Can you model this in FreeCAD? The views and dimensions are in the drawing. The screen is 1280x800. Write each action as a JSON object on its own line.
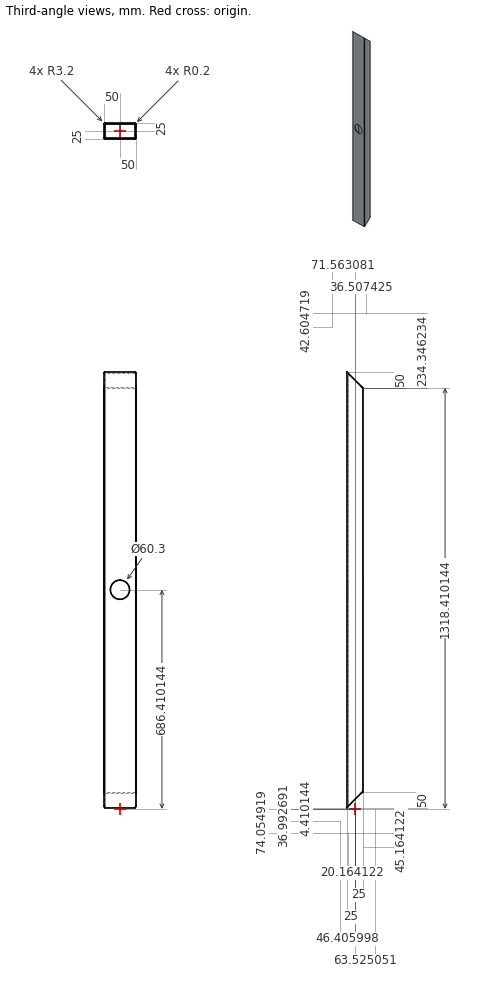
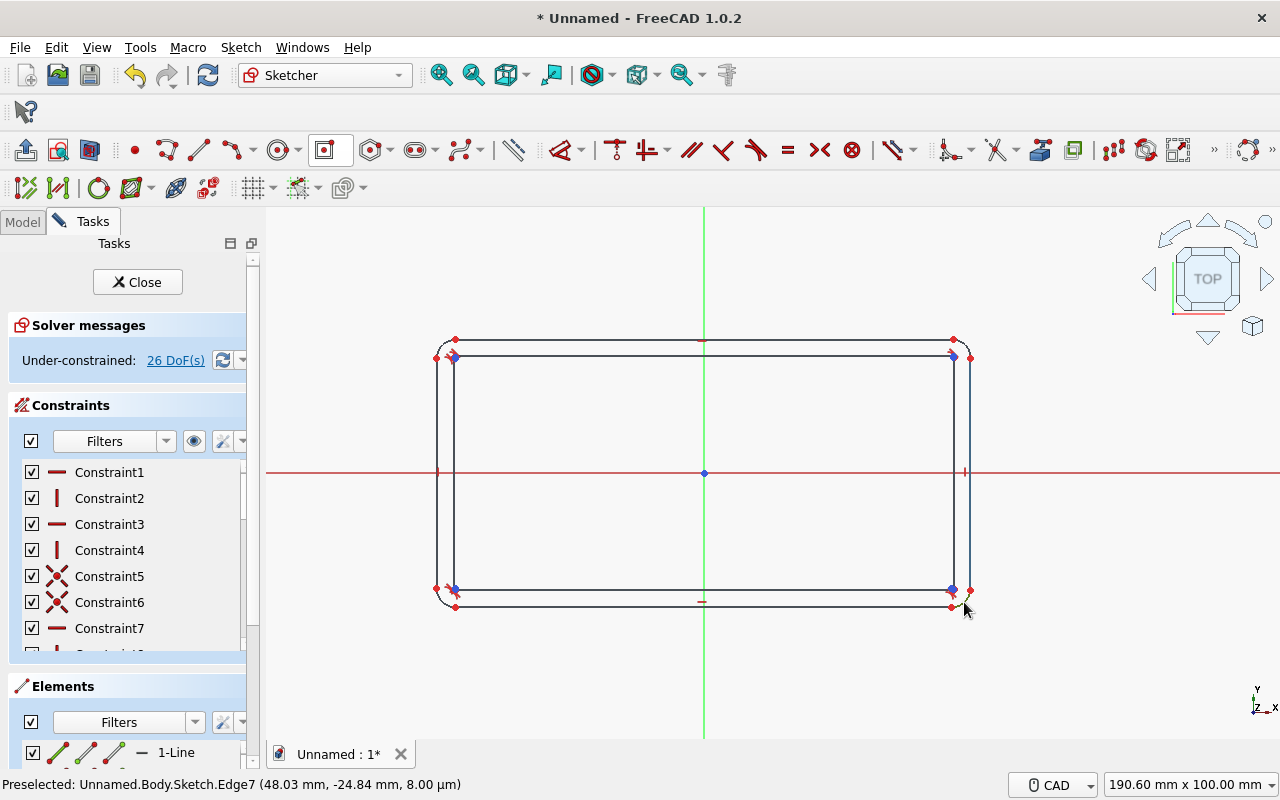
{"action": "left_click", "coordinate": [756, 150]}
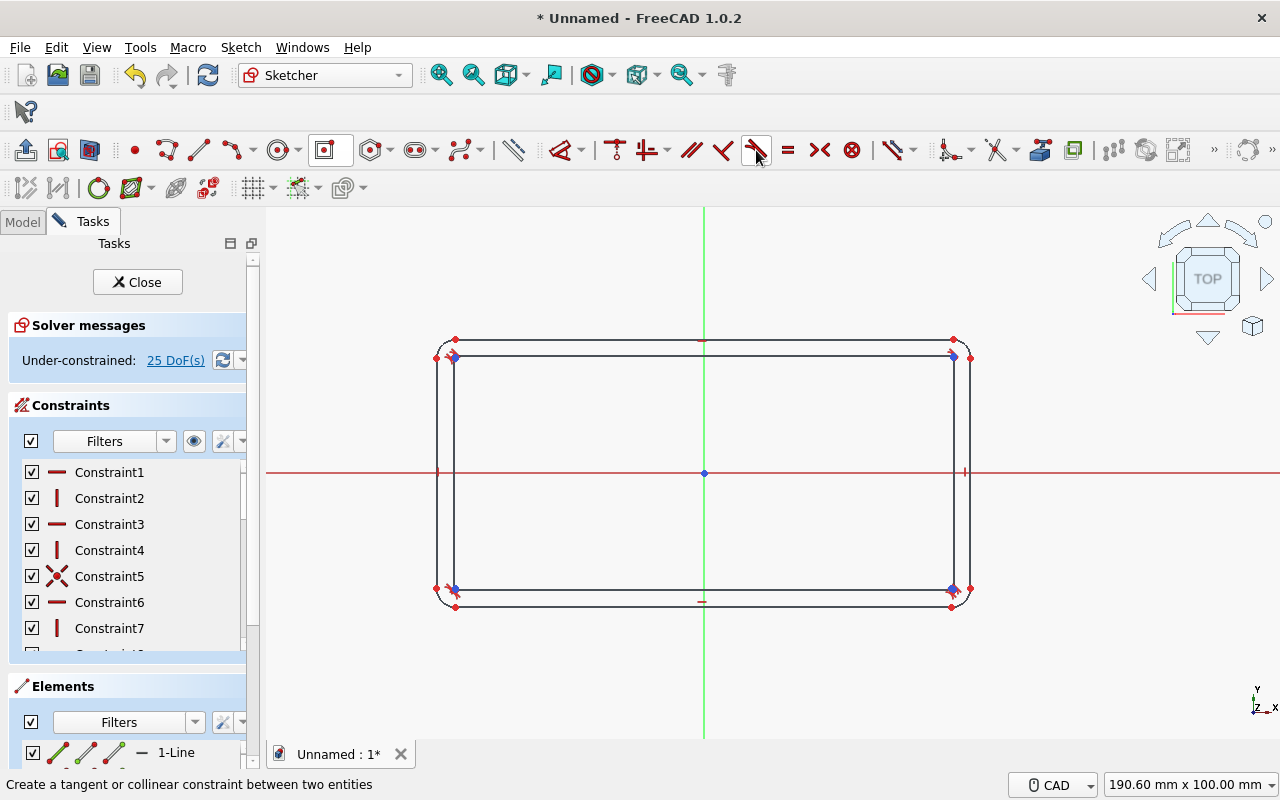
{"action": "left_click", "coordinate": [970, 520]}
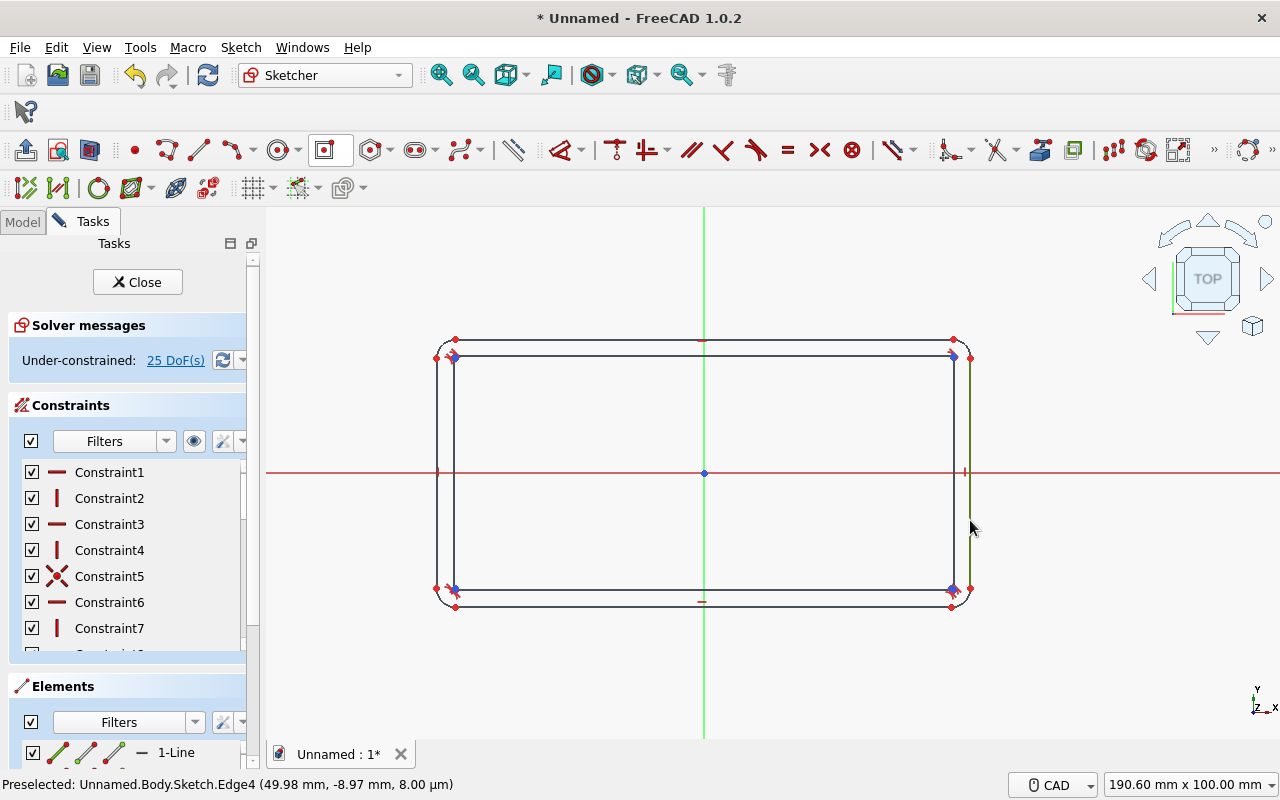
{"action": "left_click", "coordinate": [966, 345]}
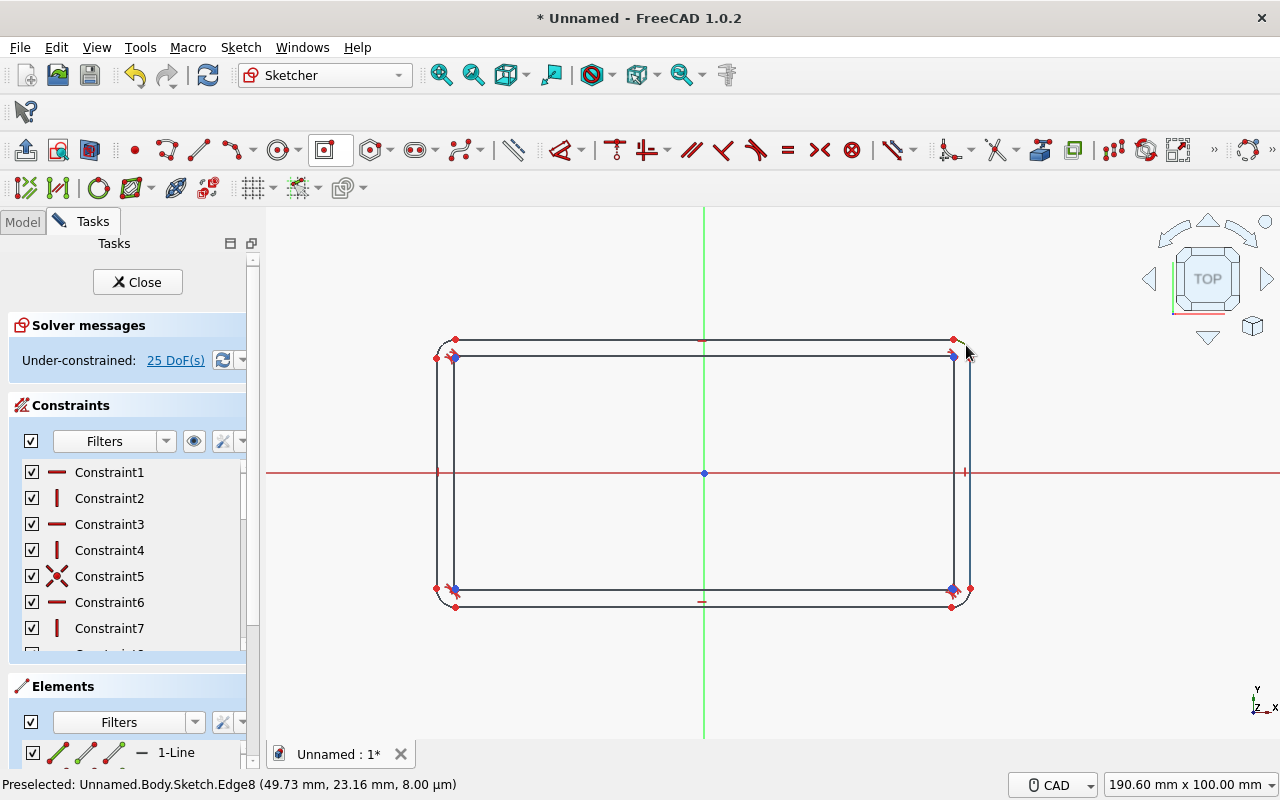
{"action": "left_click", "coordinate": [756, 150]}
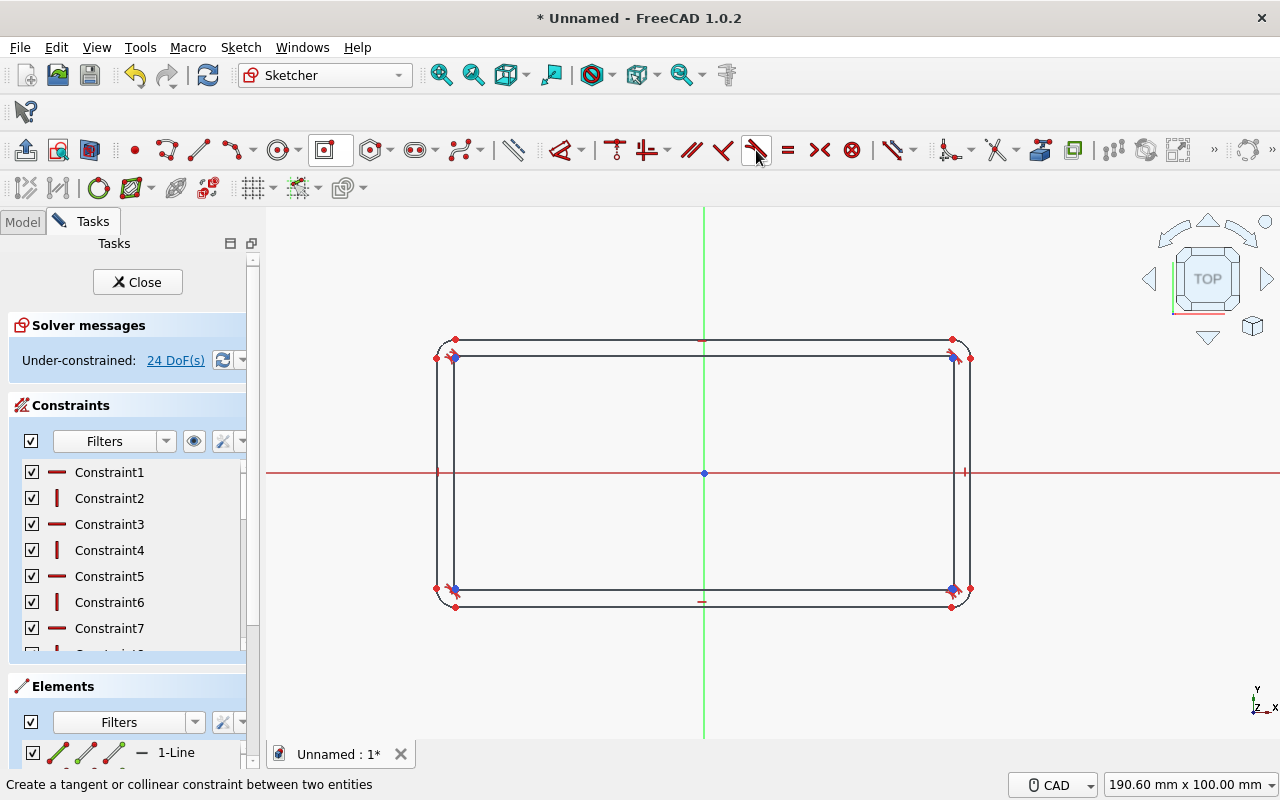
{"action": "left_click", "coordinate": [605, 356]}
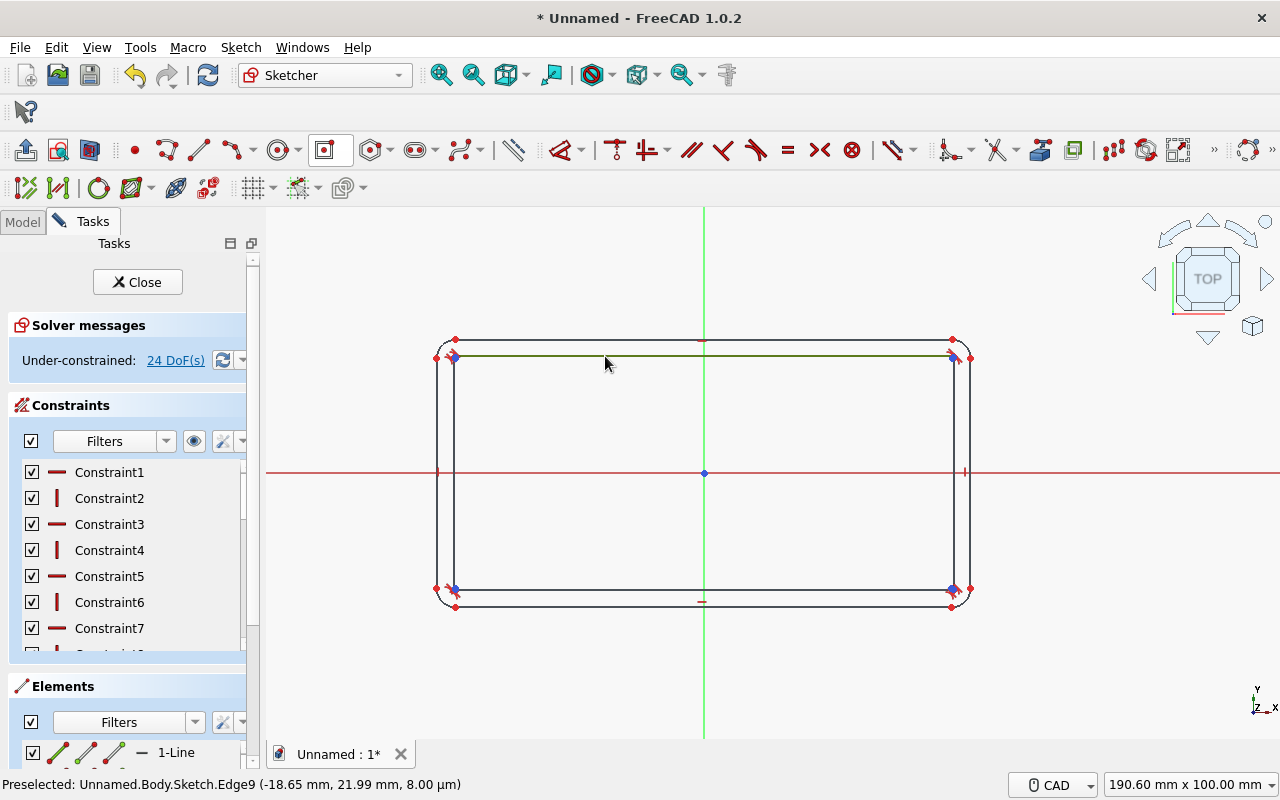
{"action": "scroll", "coordinate": [954, 357], "scroll_direction": "up", "scroll_amount": 14}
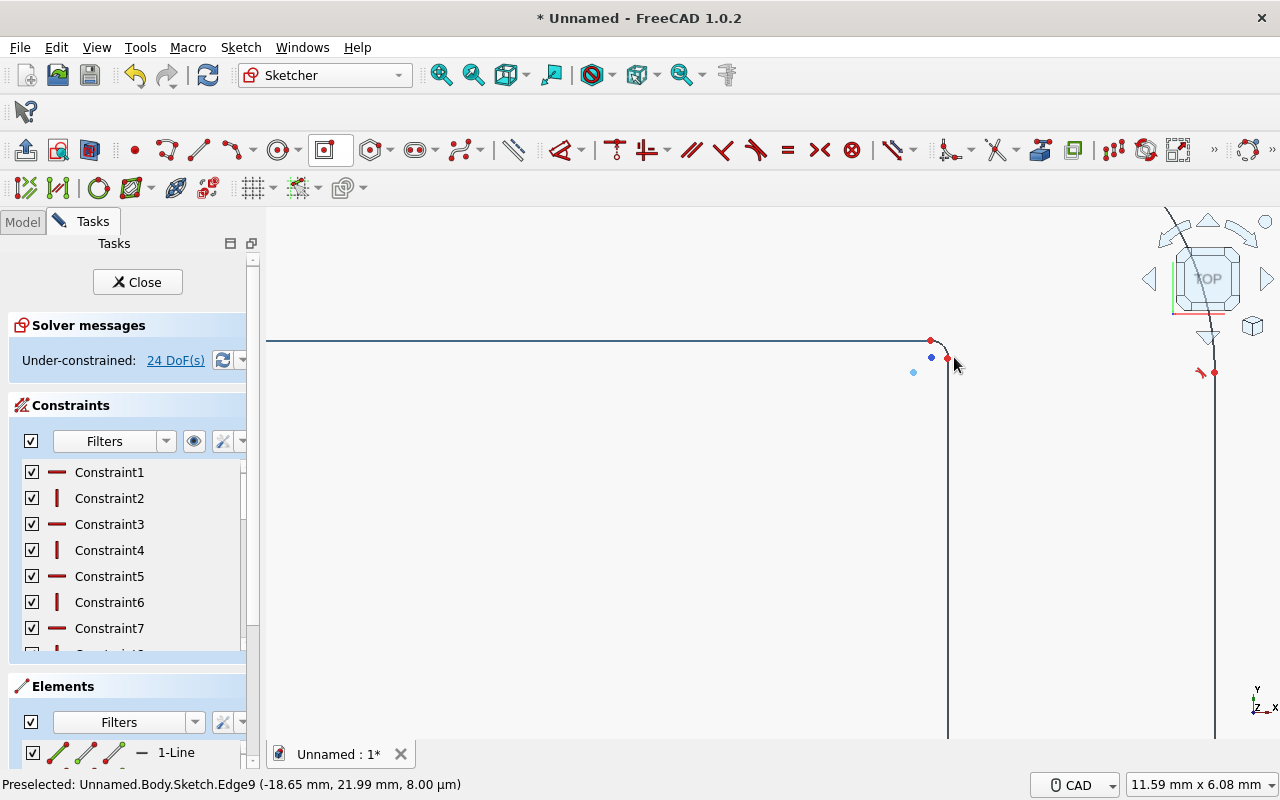
{"action": "left_click", "coordinate": [943, 346]}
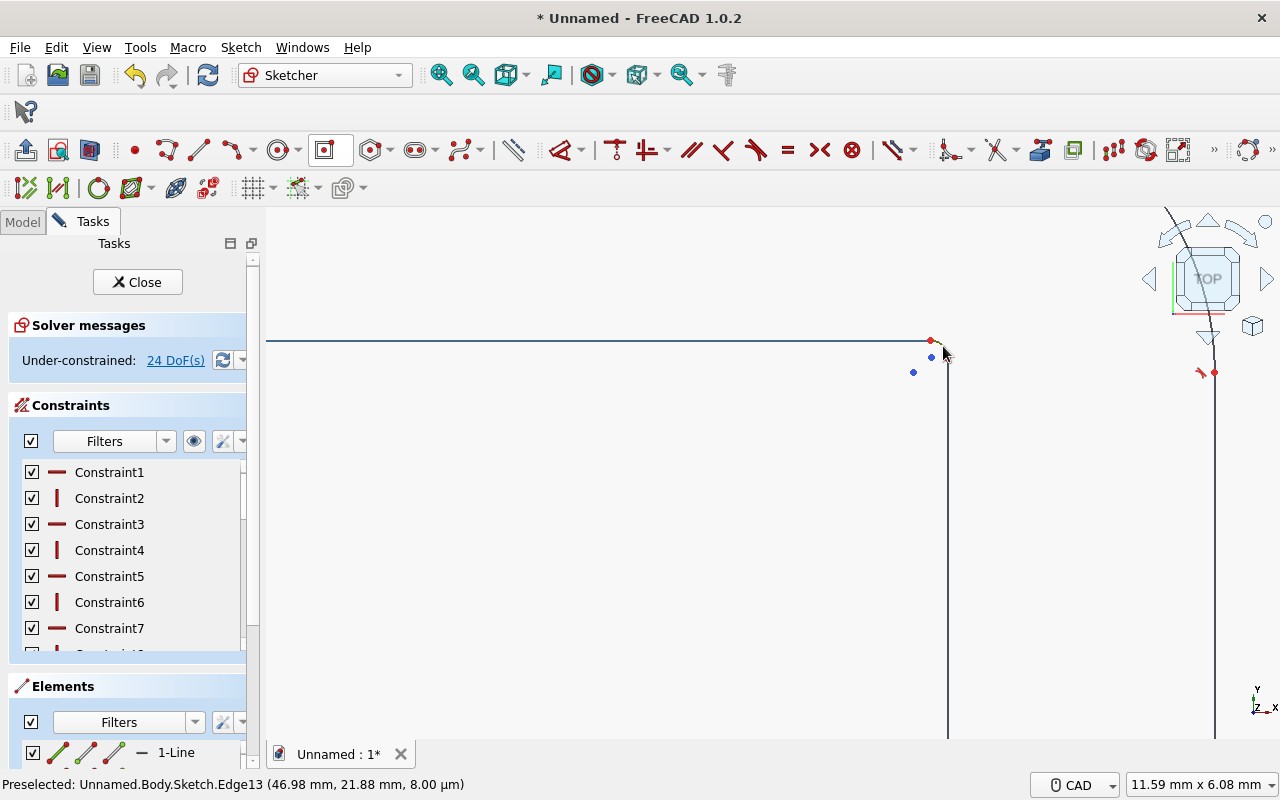
{"action": "key", "text": "t"}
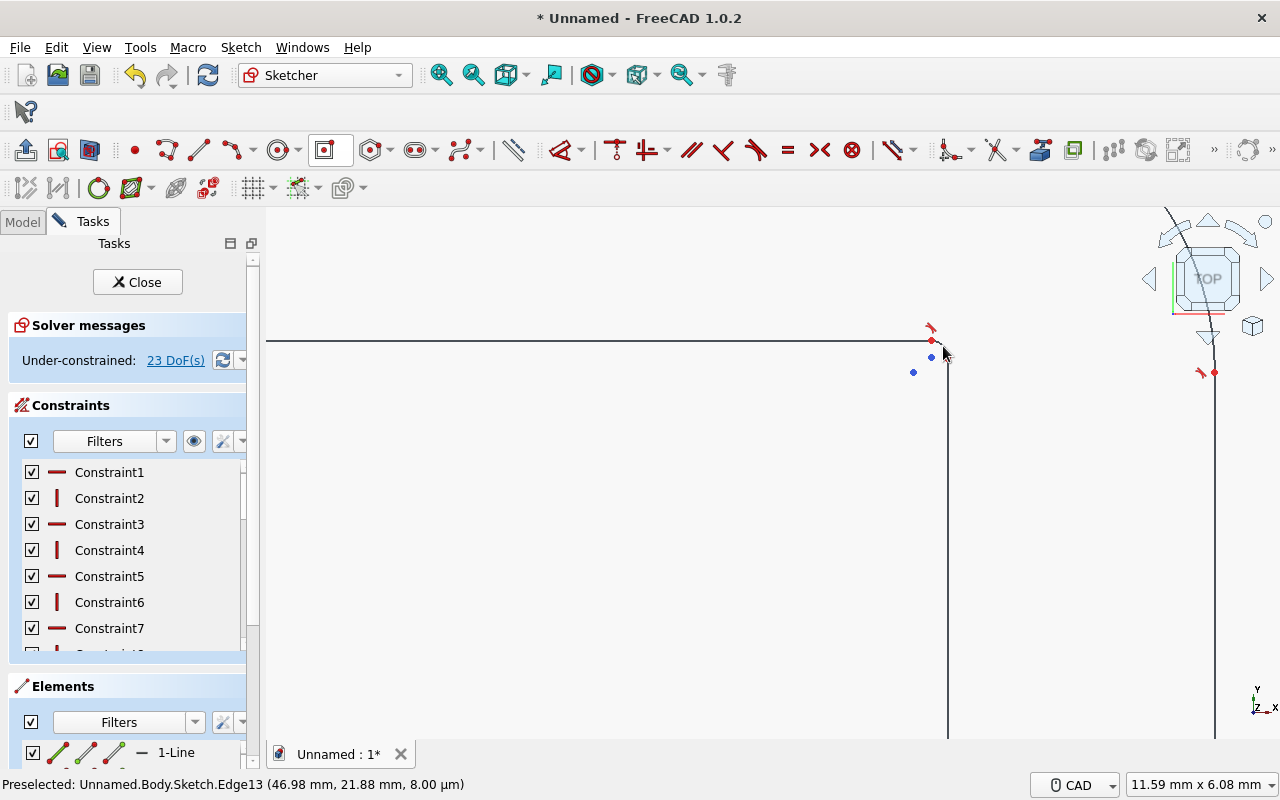
{"action": "scroll", "coordinate": [955, 357], "scroll_direction": "down", "scroll_amount": 14}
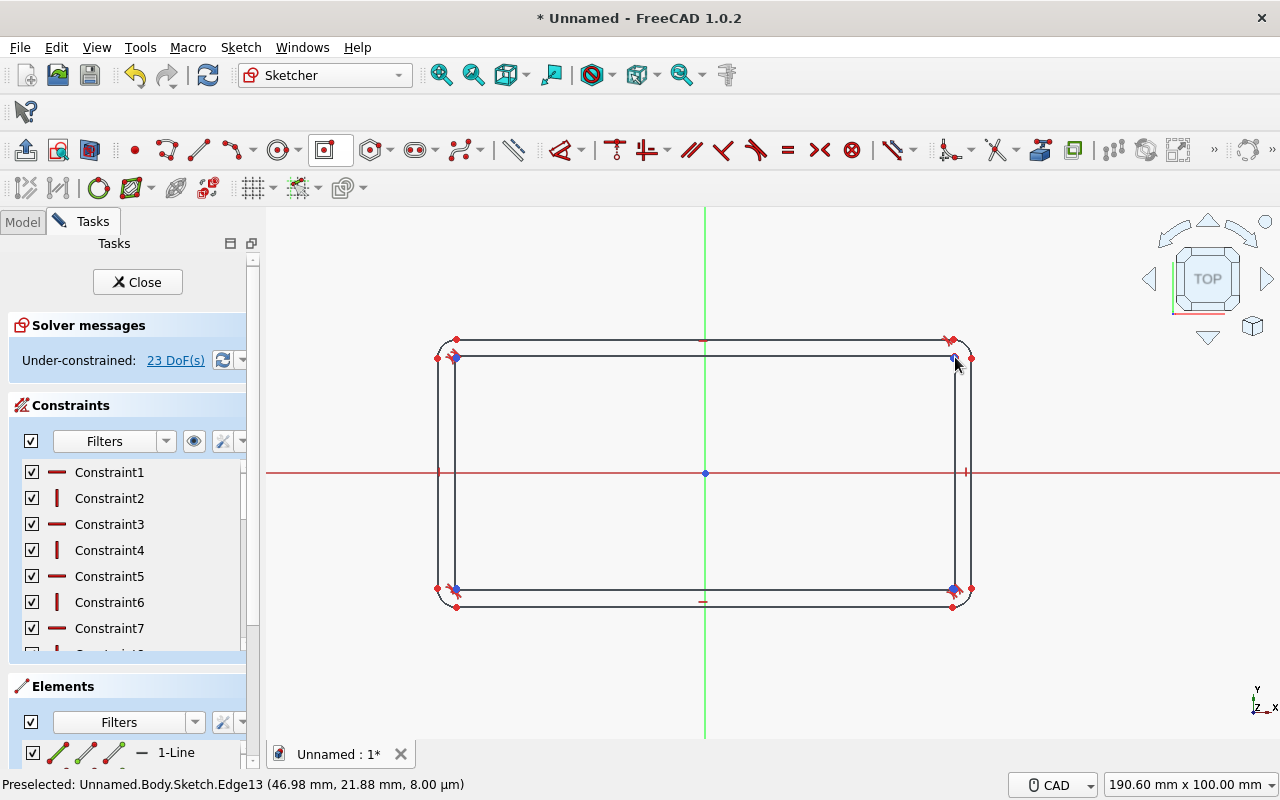
{"action": "left_click", "coordinate": [606, 356]}